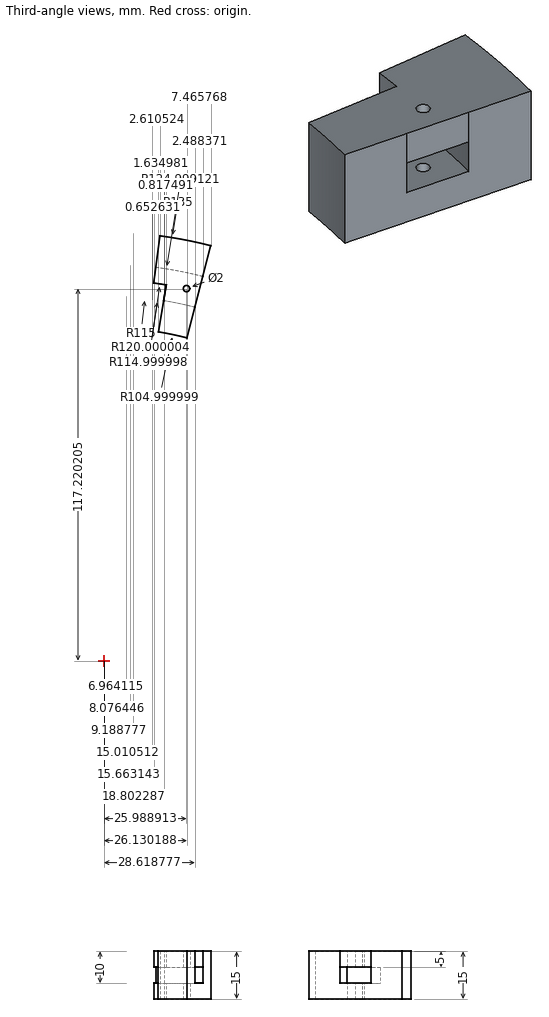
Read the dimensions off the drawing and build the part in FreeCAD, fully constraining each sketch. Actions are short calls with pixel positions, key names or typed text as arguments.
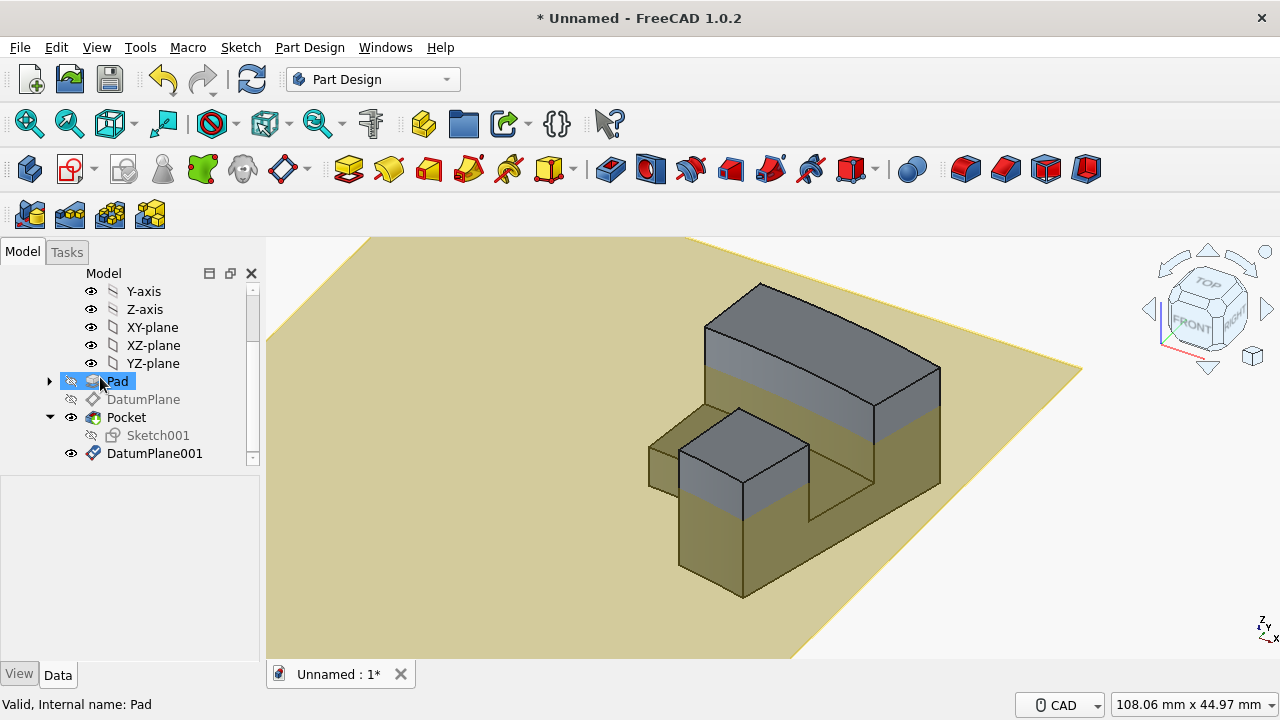
click(116, 453)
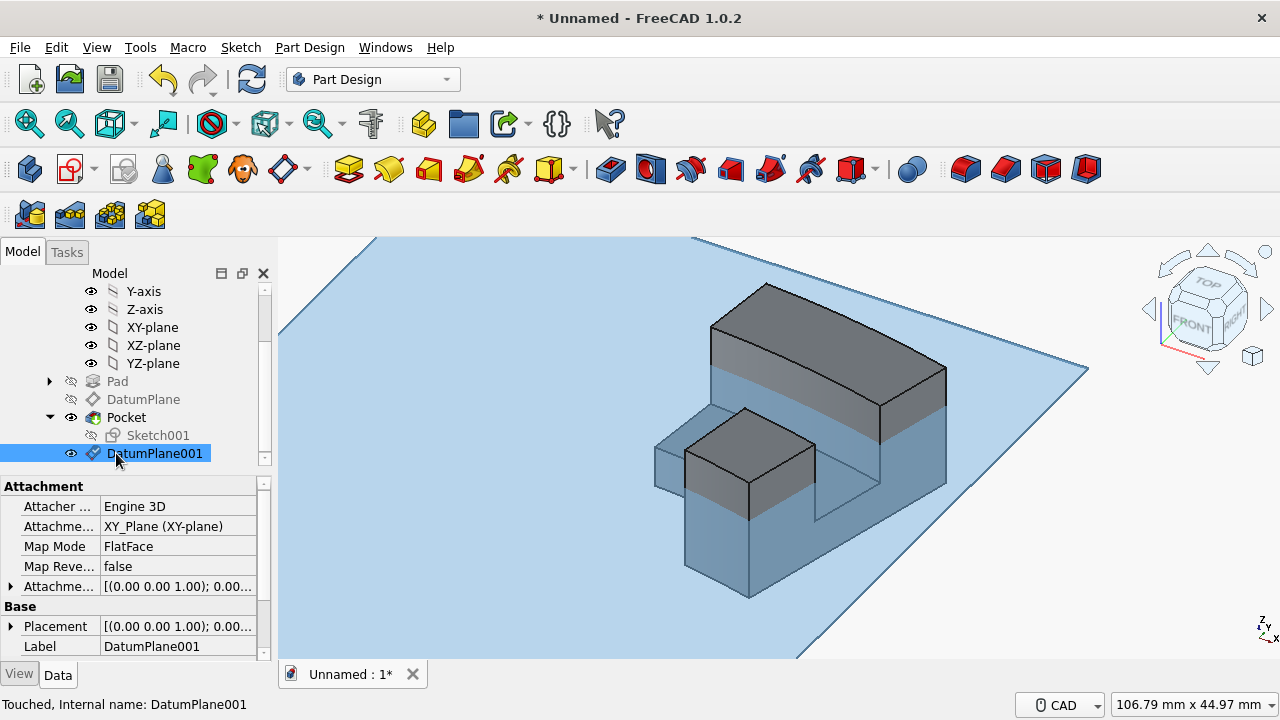
click(70, 170)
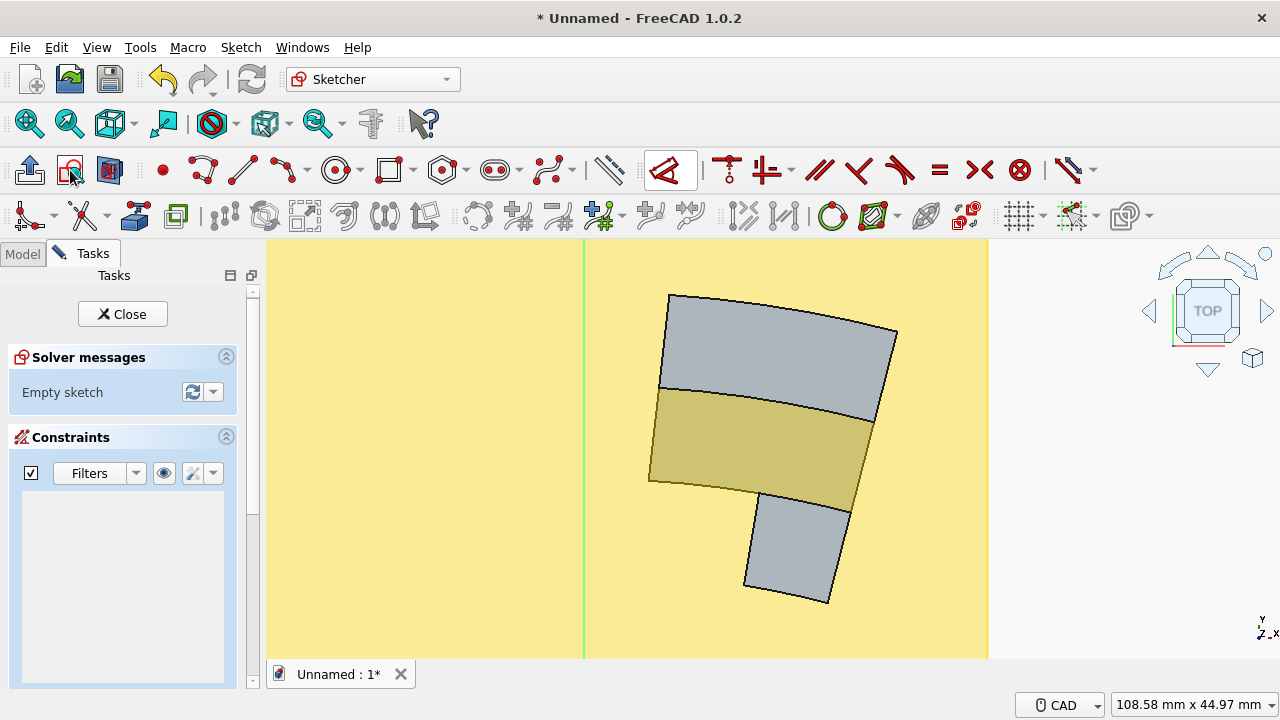
click(110, 170)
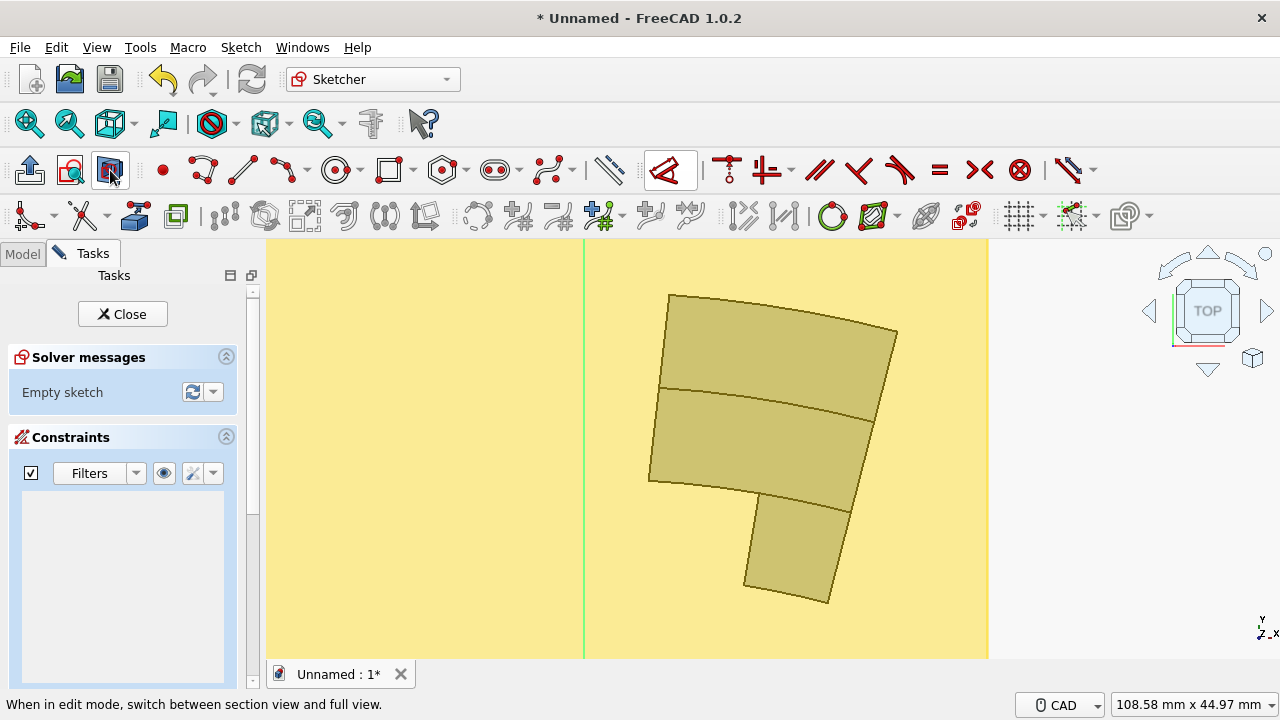
scroll(808, 451, up, 4)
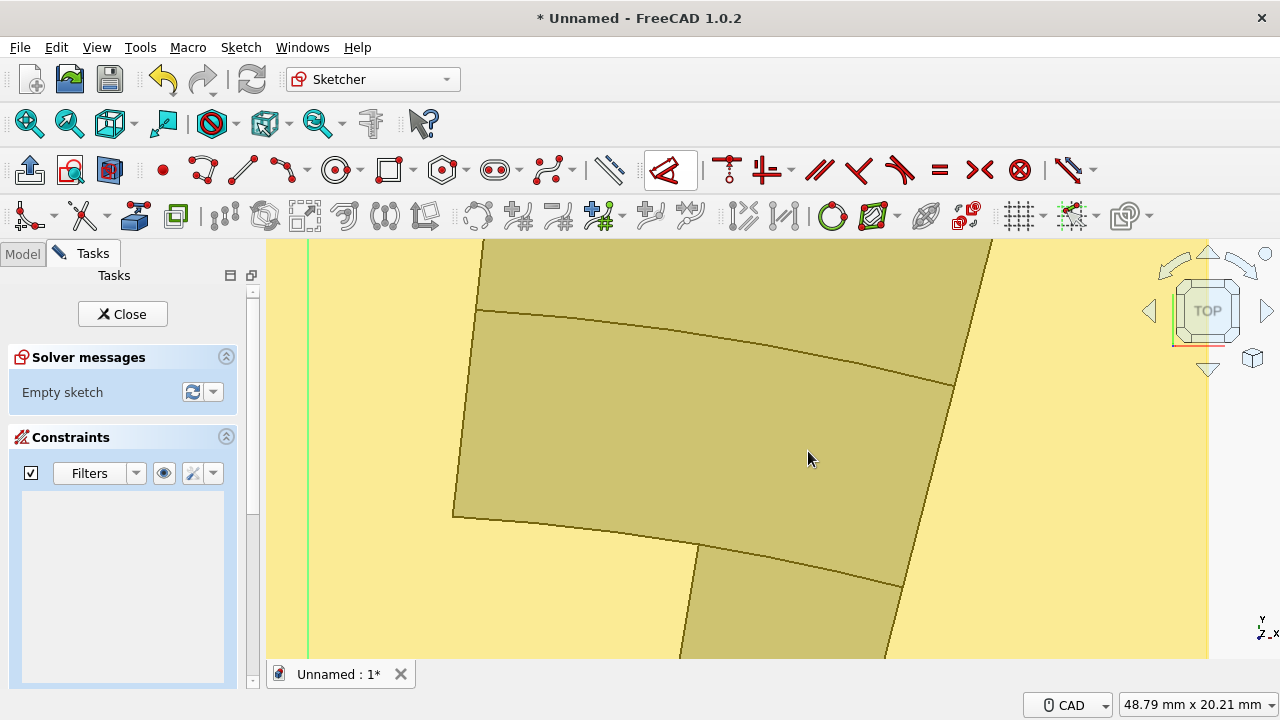
click(244, 170)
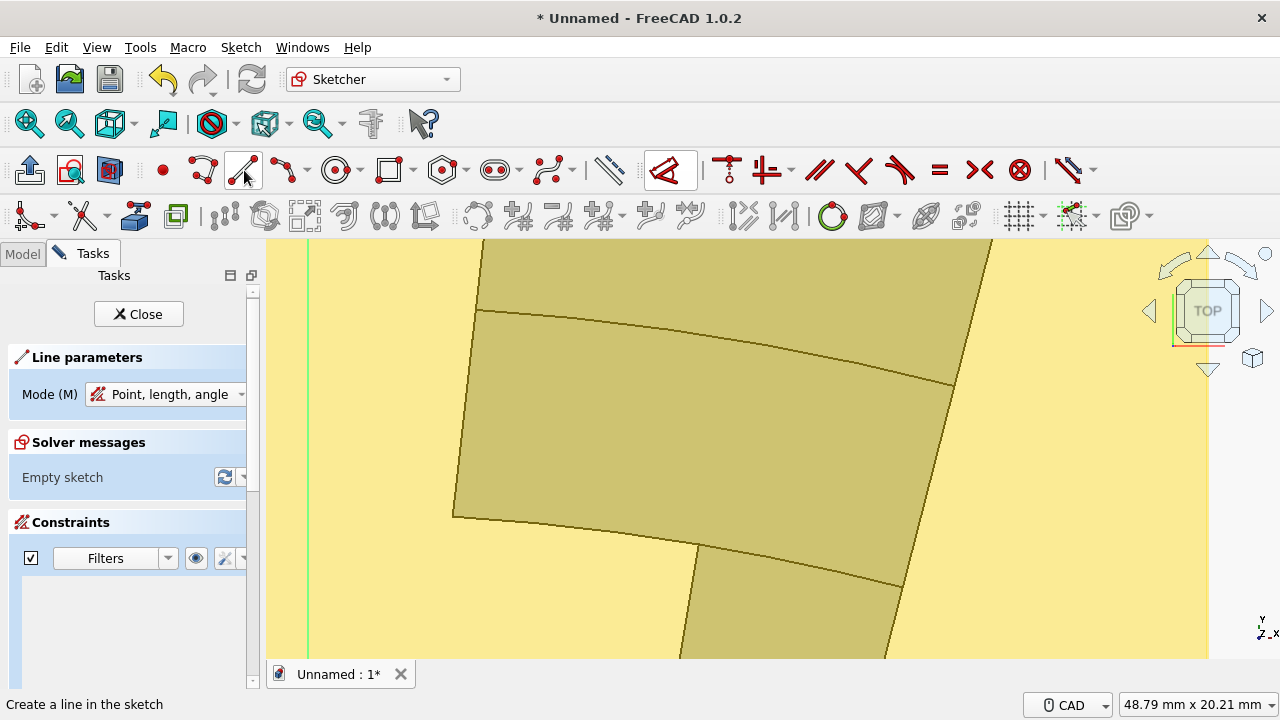
click(903, 587)
click(954, 386)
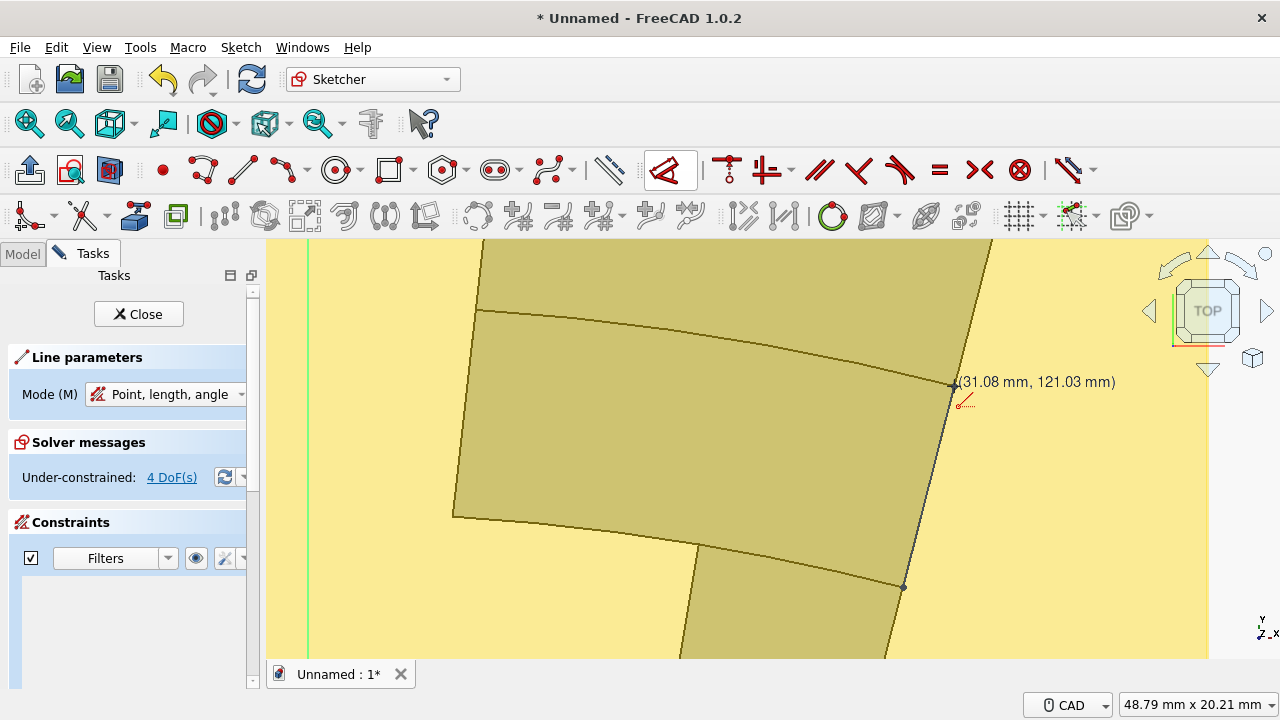
click(476, 310)
click(453, 517)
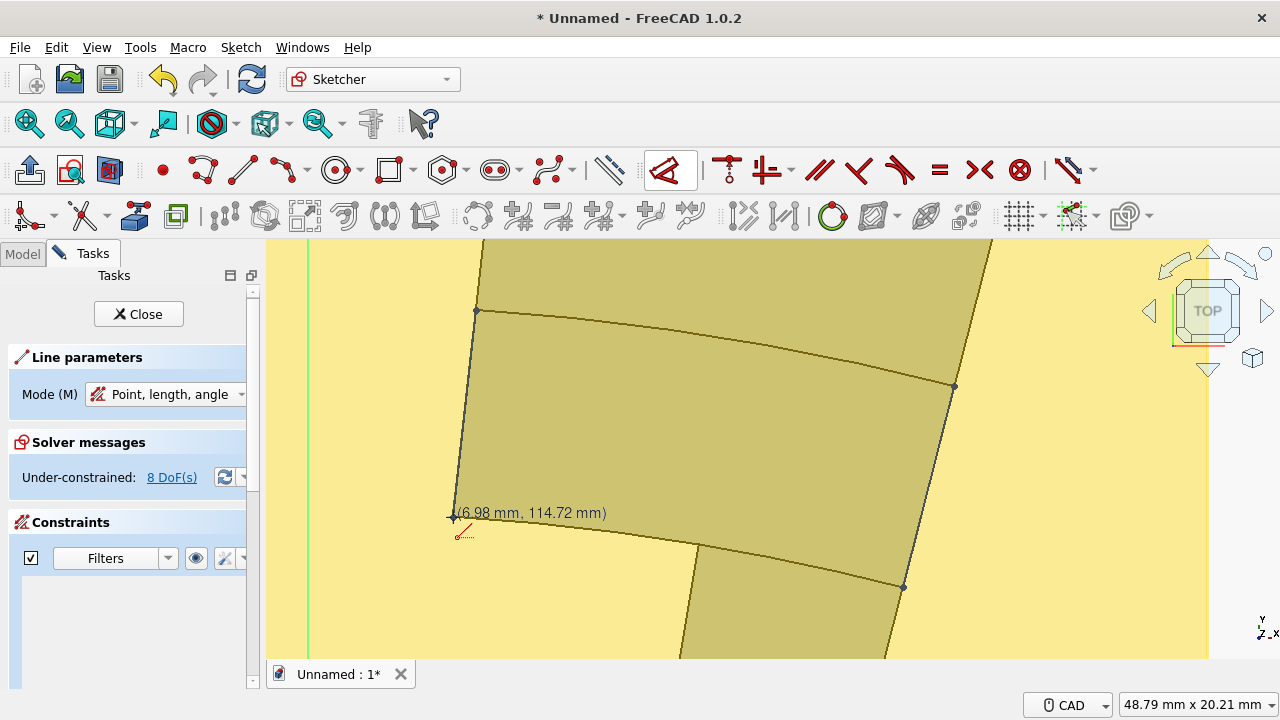
click(284, 170)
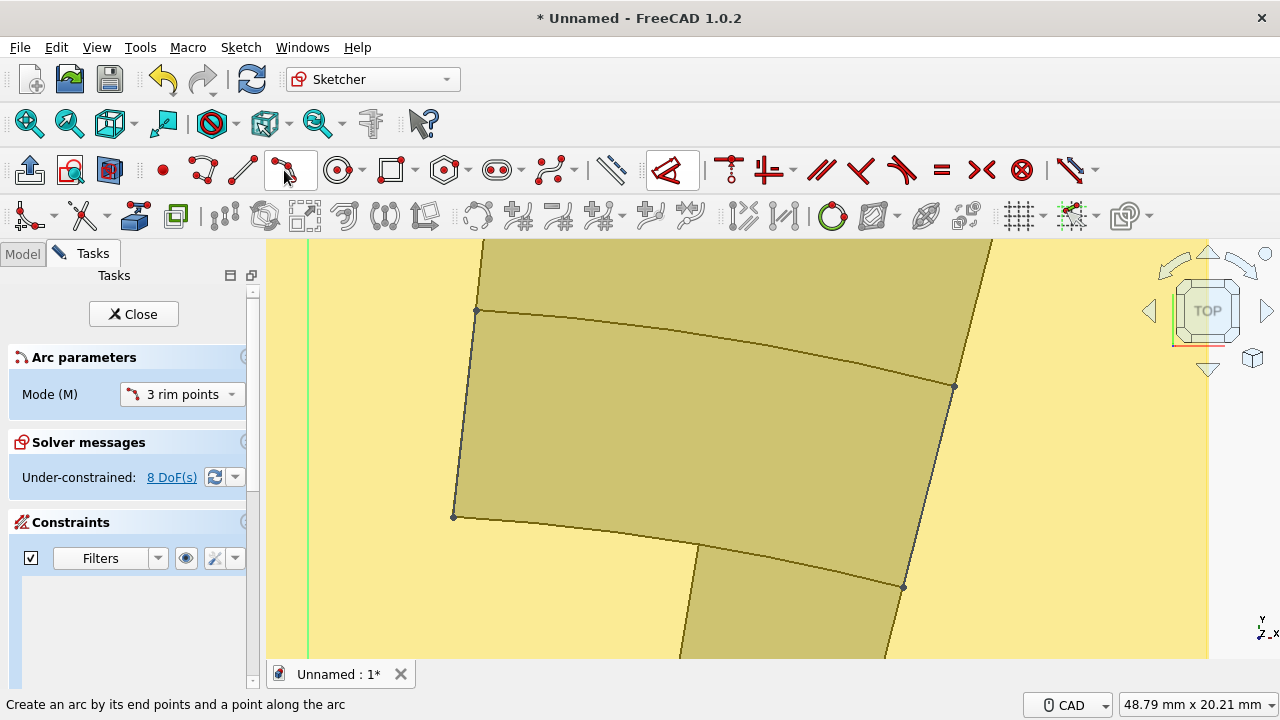
click(954, 387)
click(476, 311)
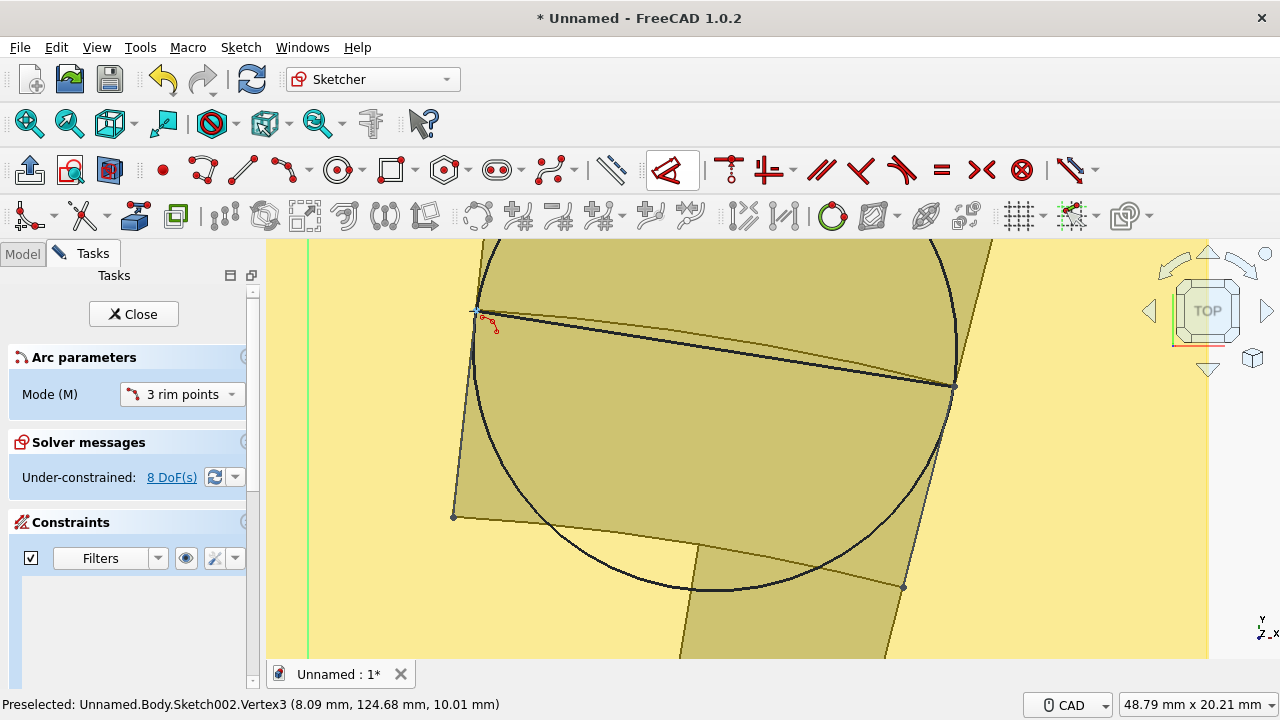
scroll(717, 337, up, 2)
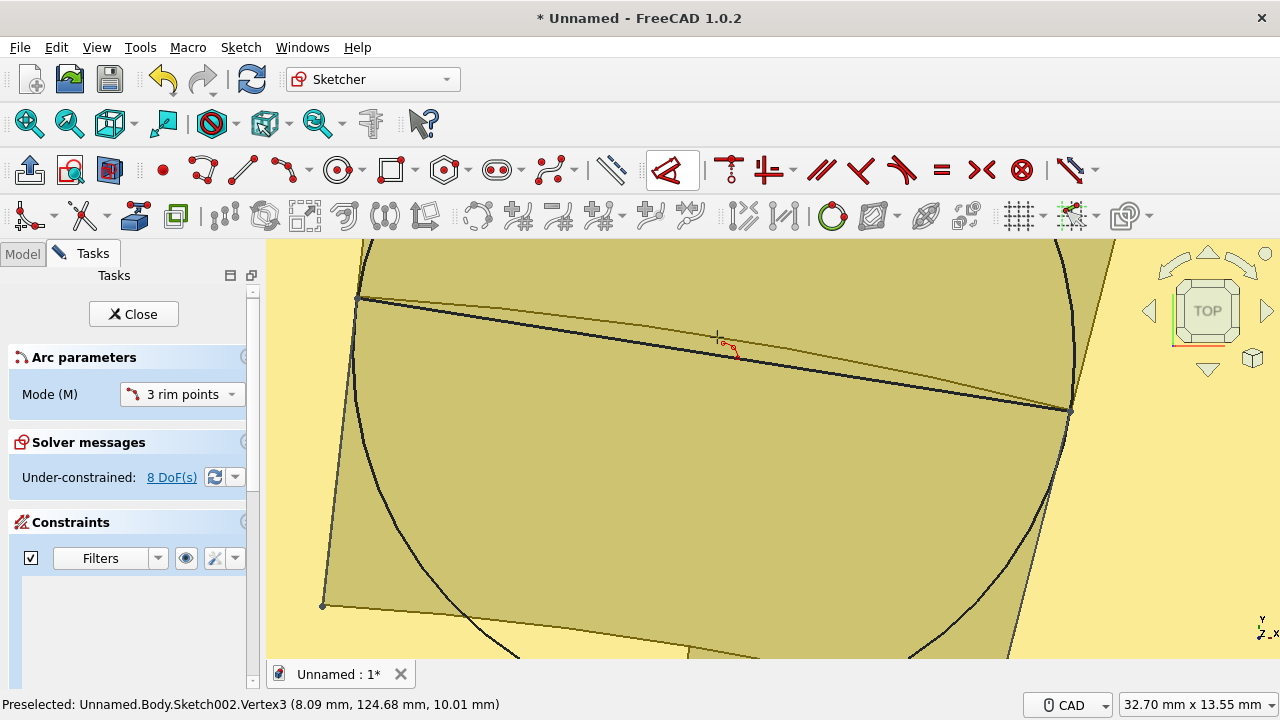
click(717, 337)